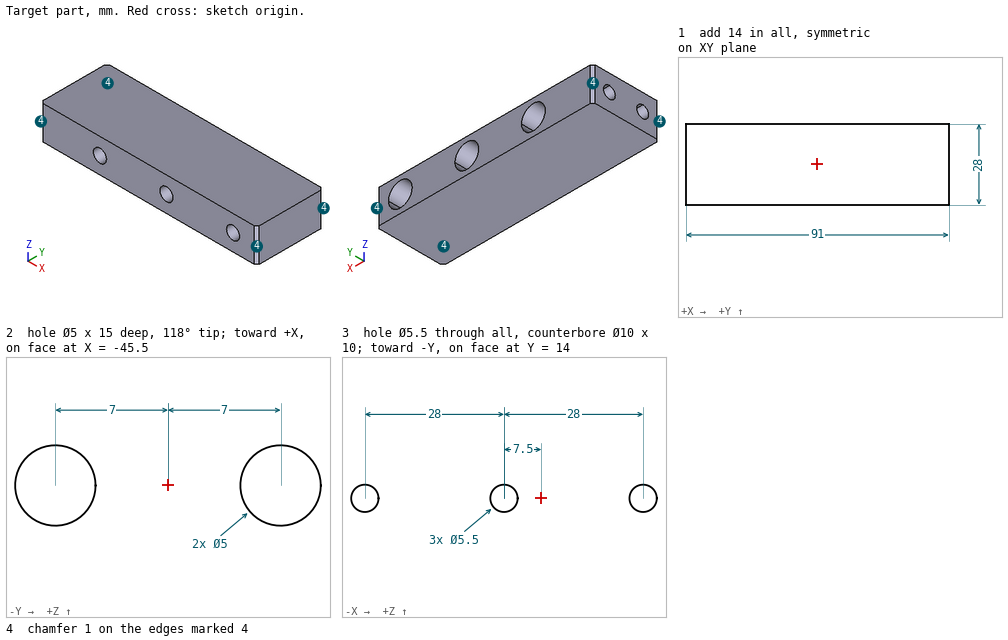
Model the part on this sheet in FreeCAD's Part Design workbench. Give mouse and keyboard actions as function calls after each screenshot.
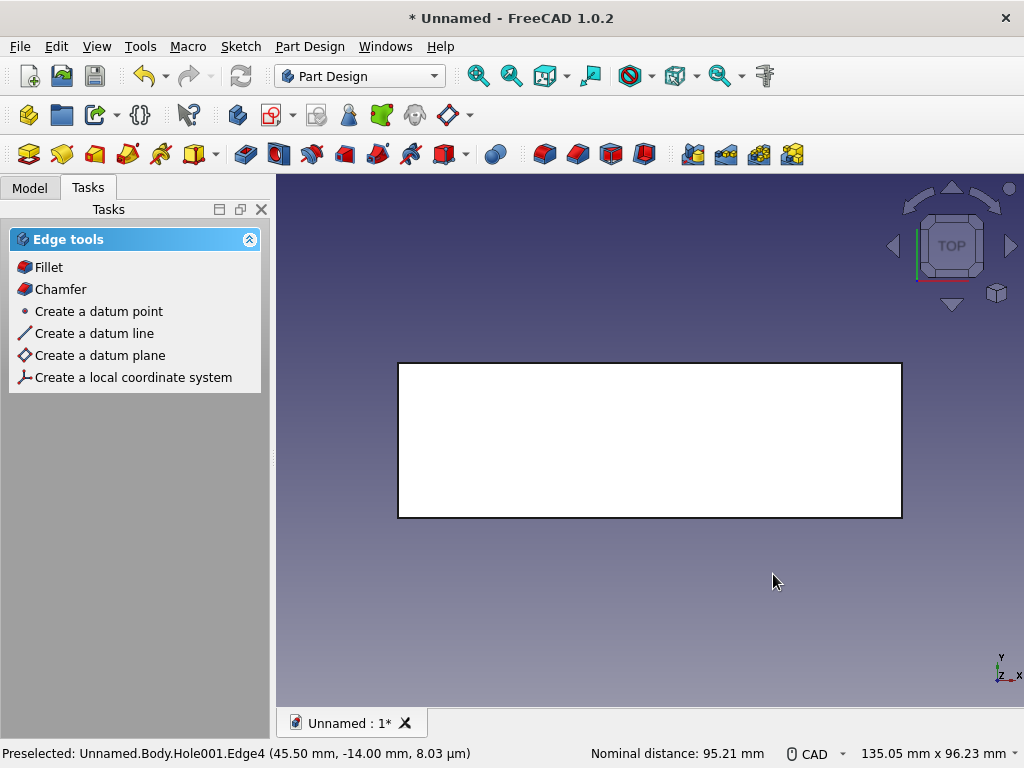
key(1)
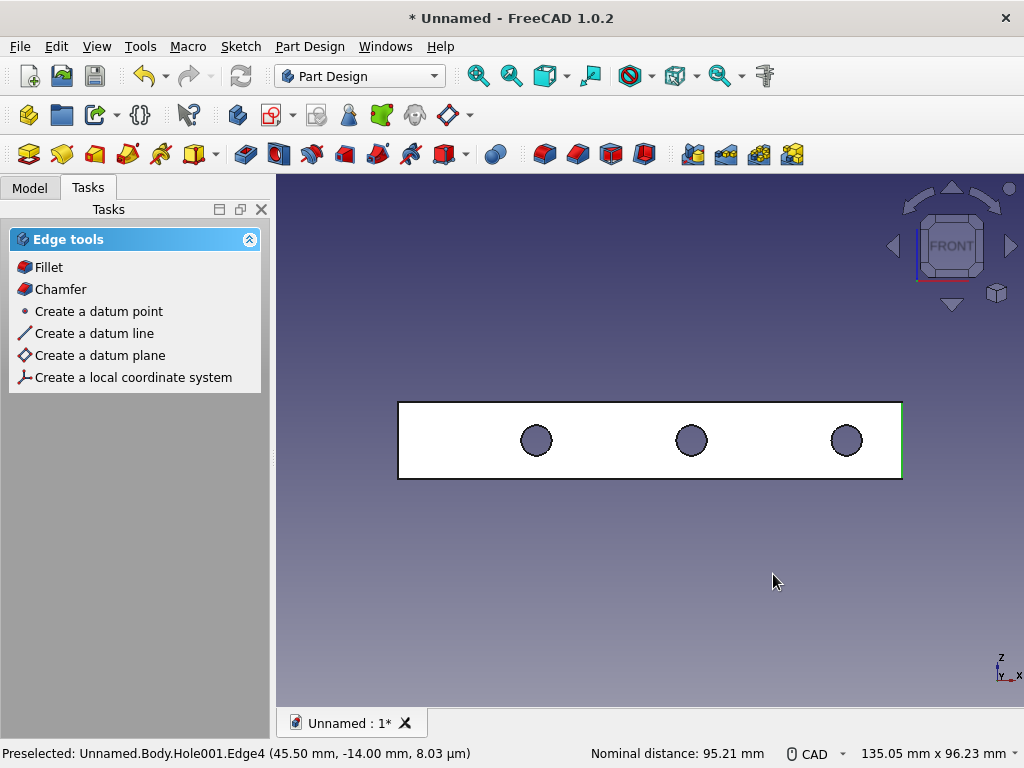
click(398, 440, ctrl)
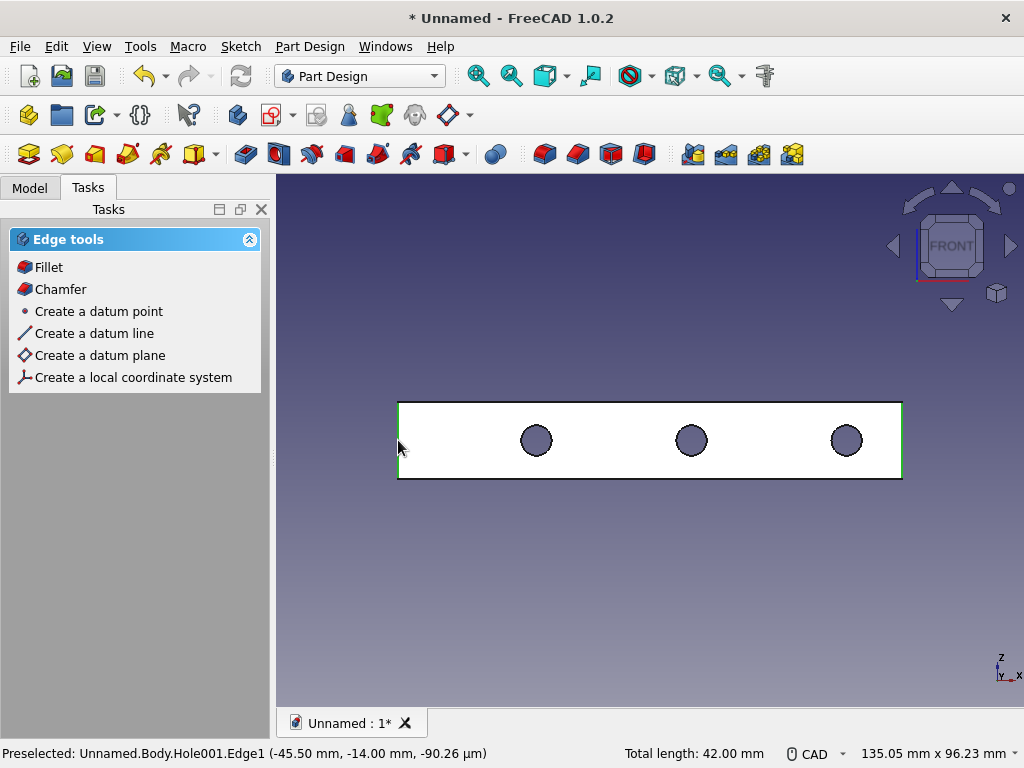
key(3)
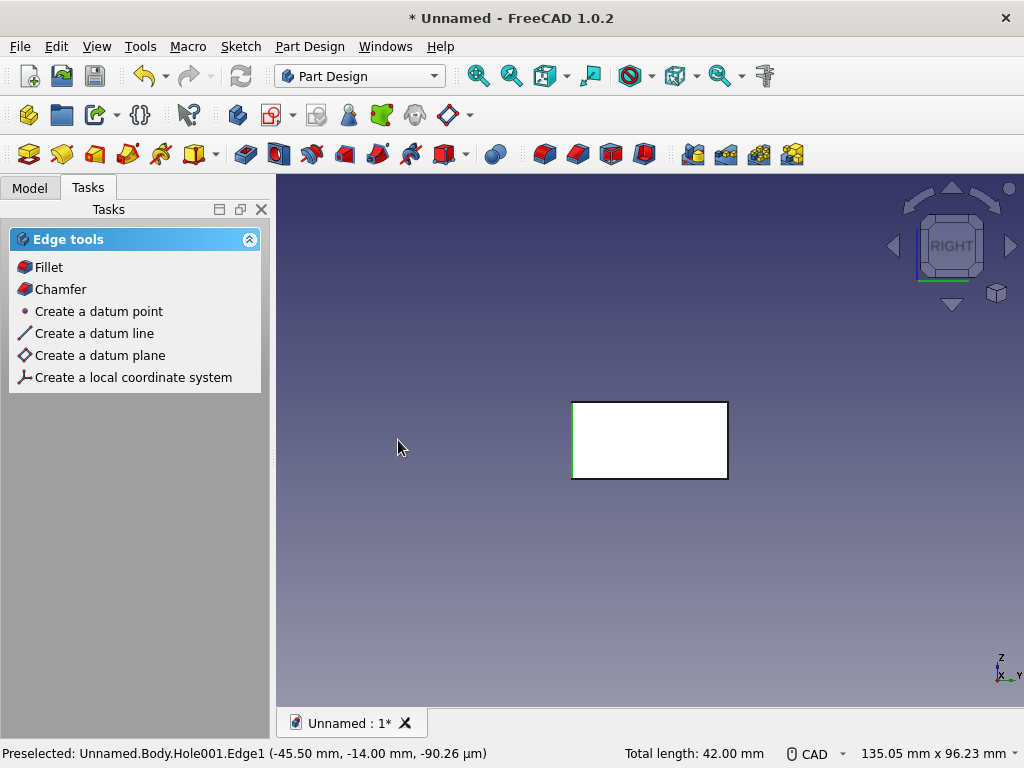
click(479, 76)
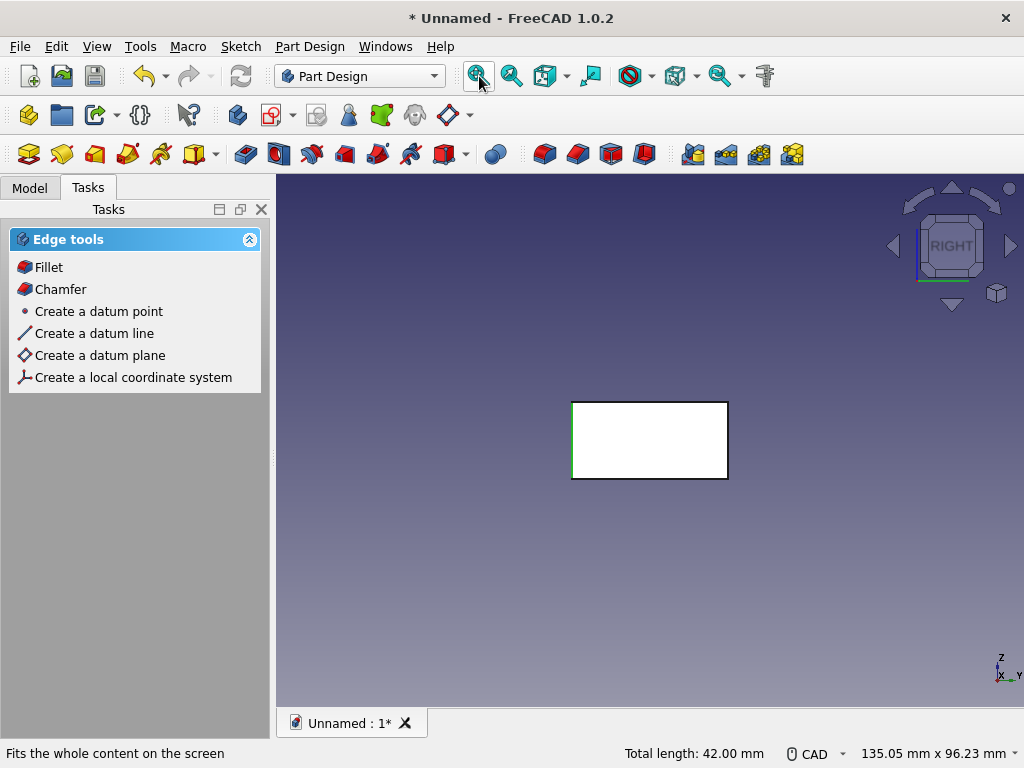
click(728, 439, ctrl)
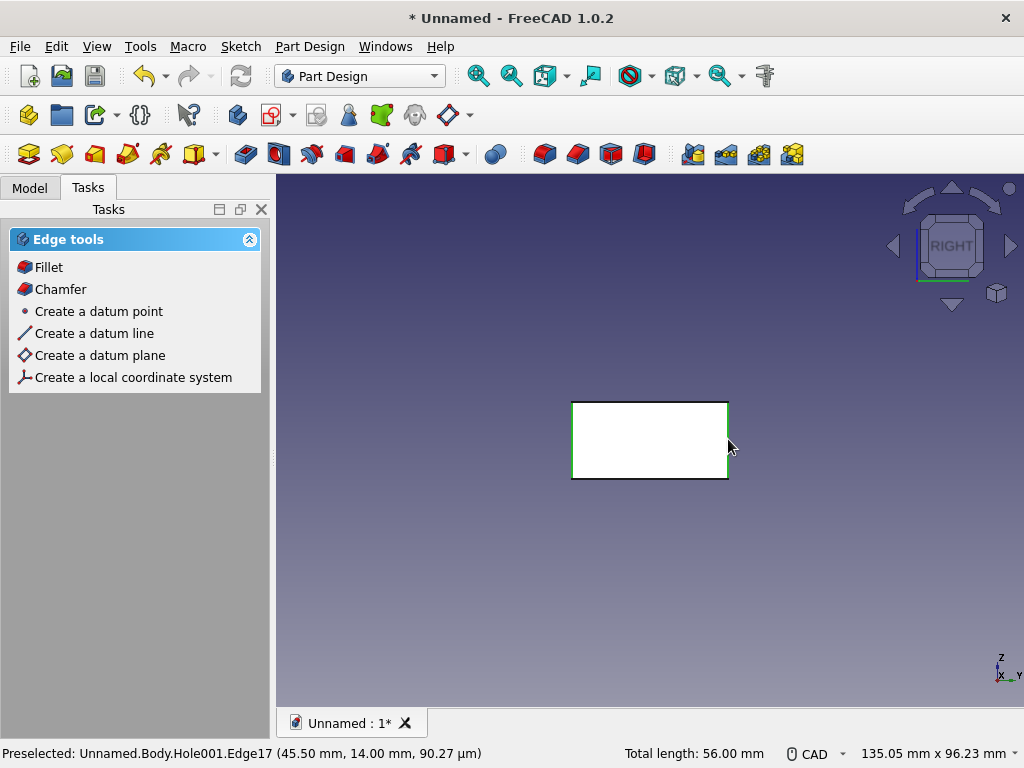
click(578, 154)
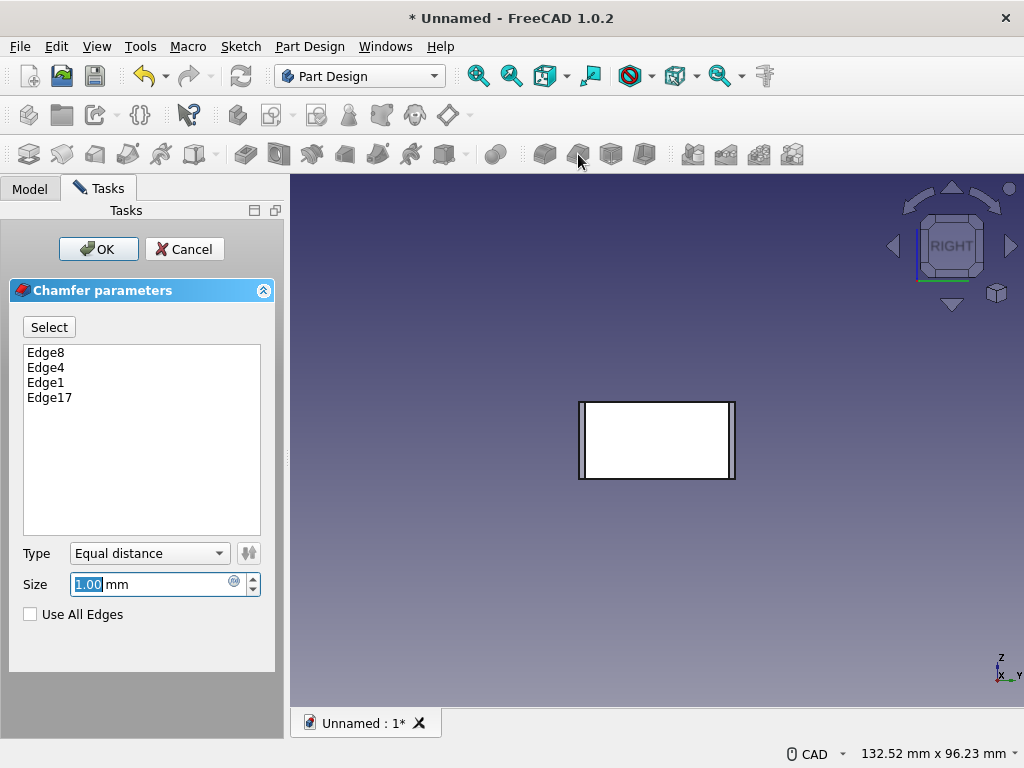
text(1)
key(Tab)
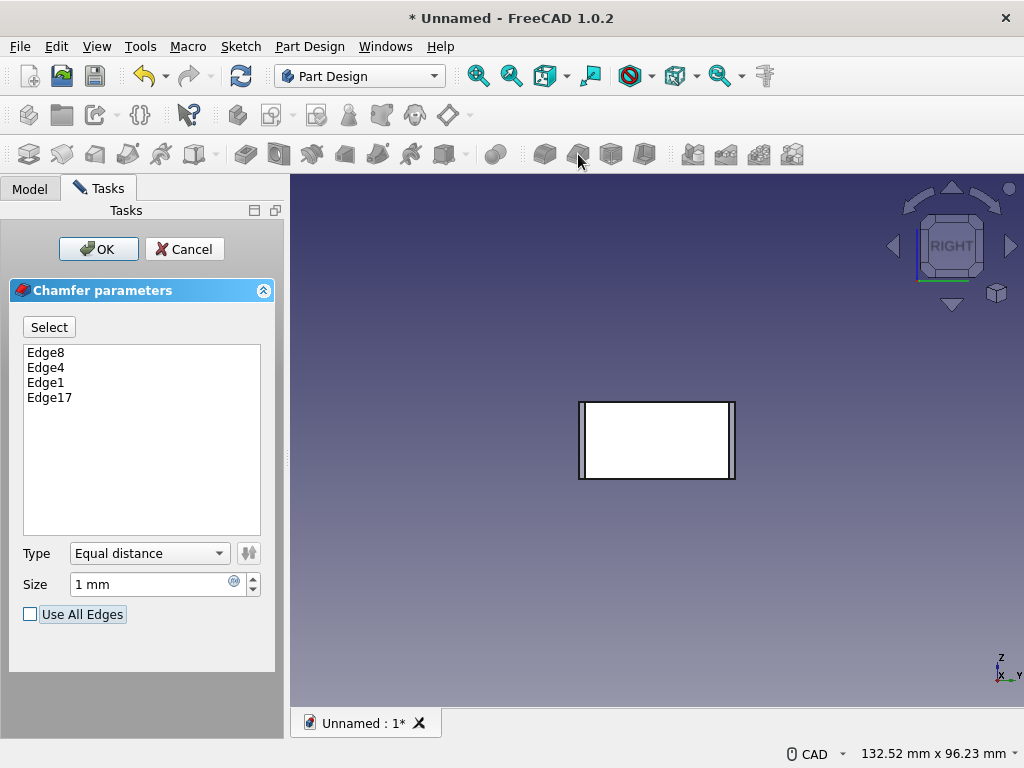
click(99, 249)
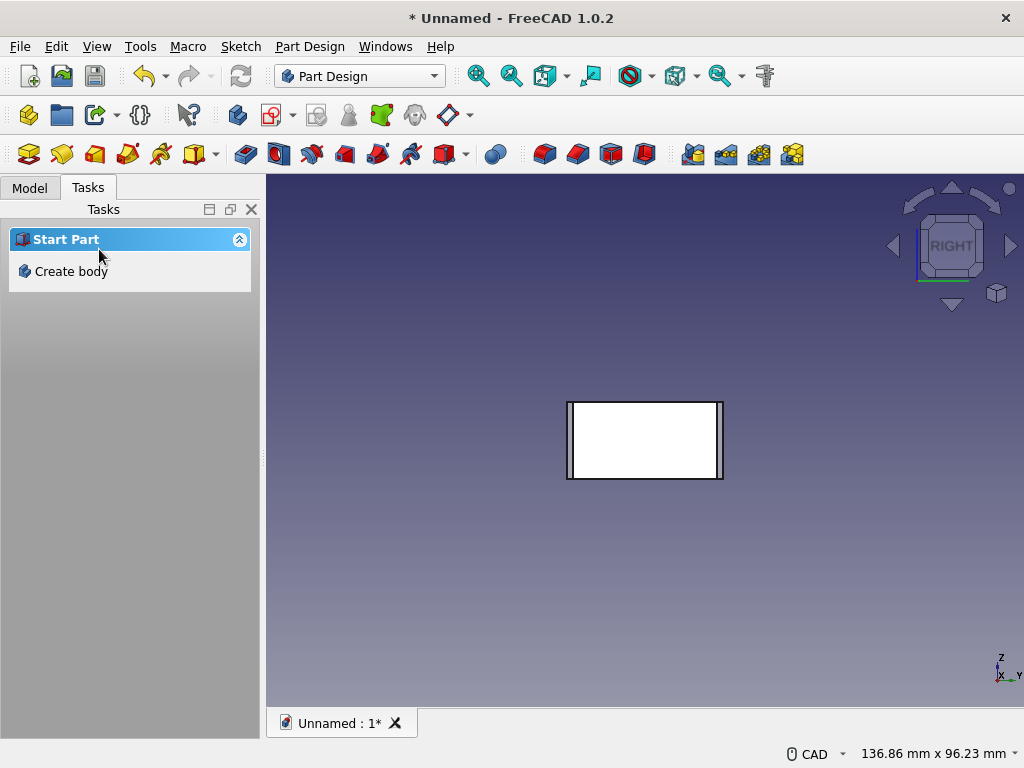
key(0)